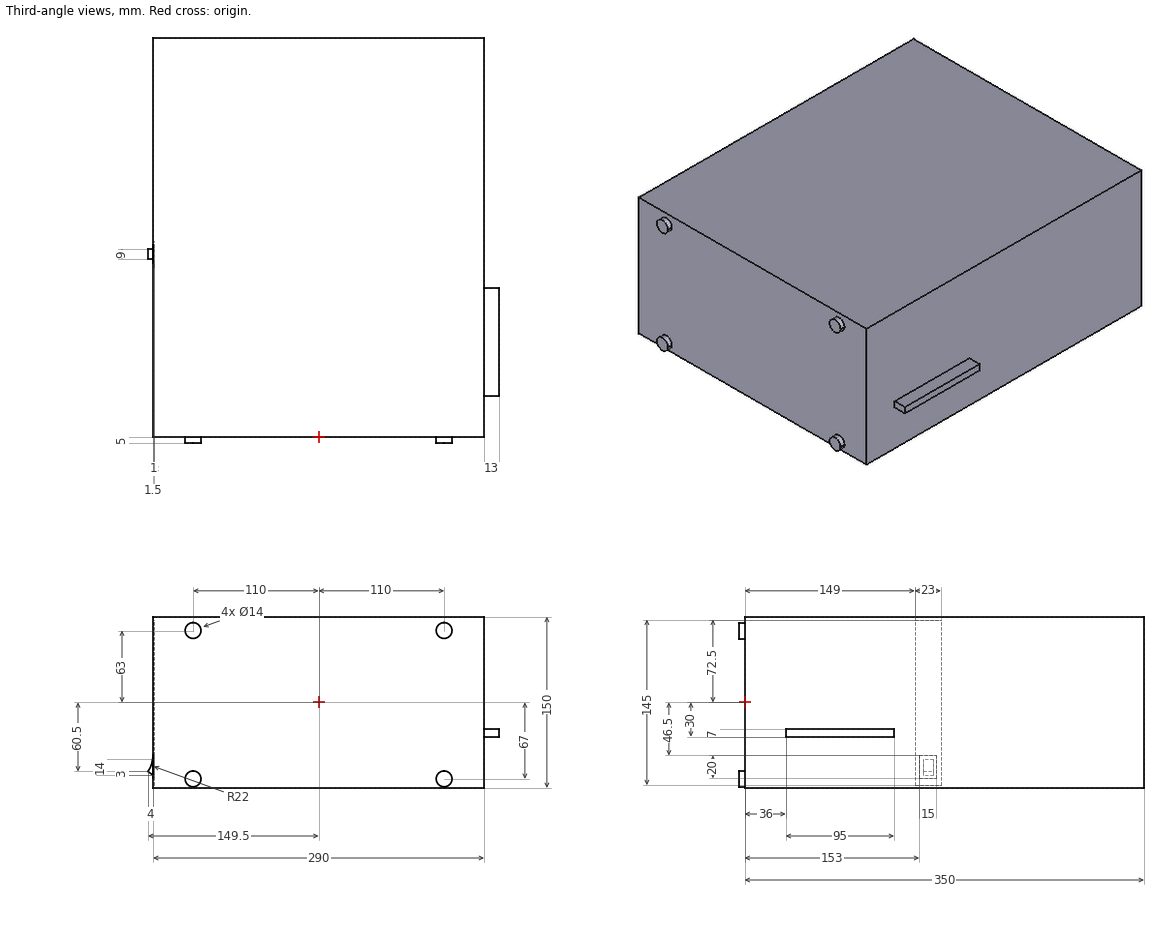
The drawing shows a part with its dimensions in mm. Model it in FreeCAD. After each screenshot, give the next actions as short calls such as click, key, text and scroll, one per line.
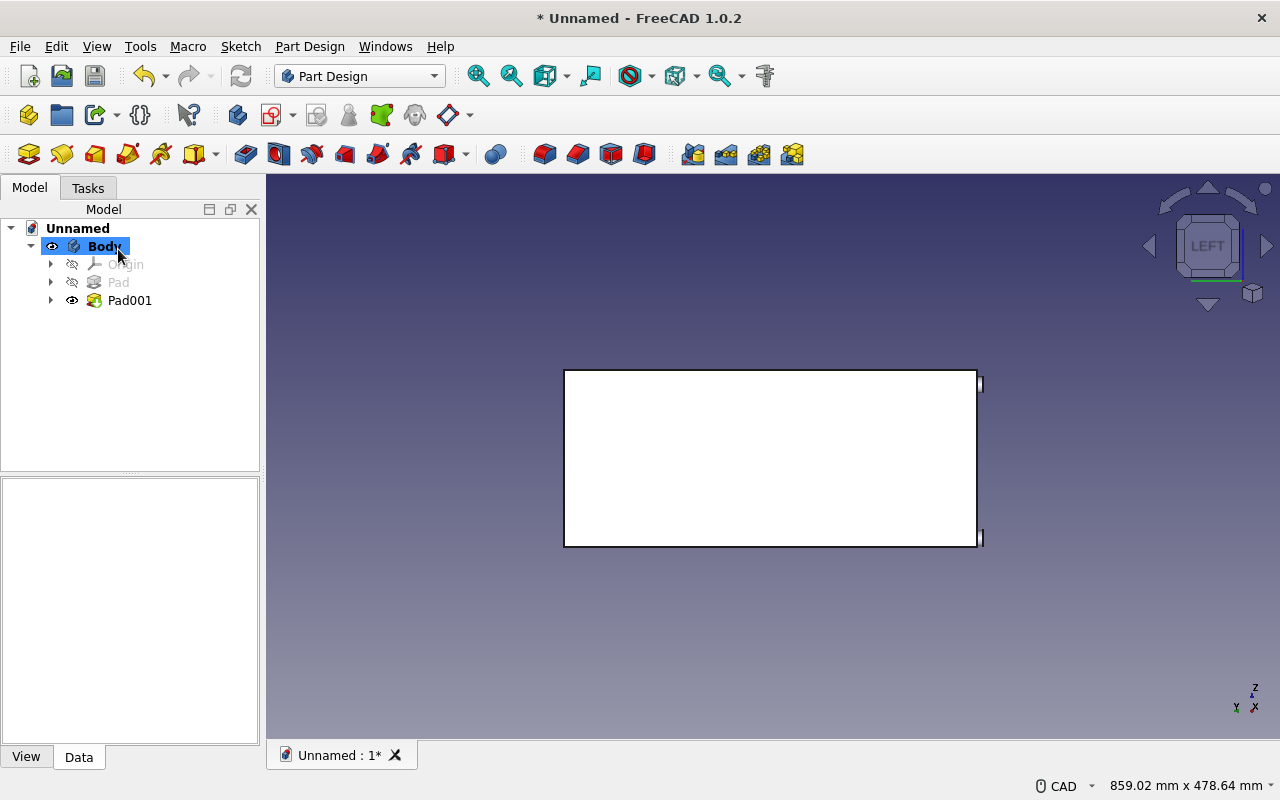
click(479, 76)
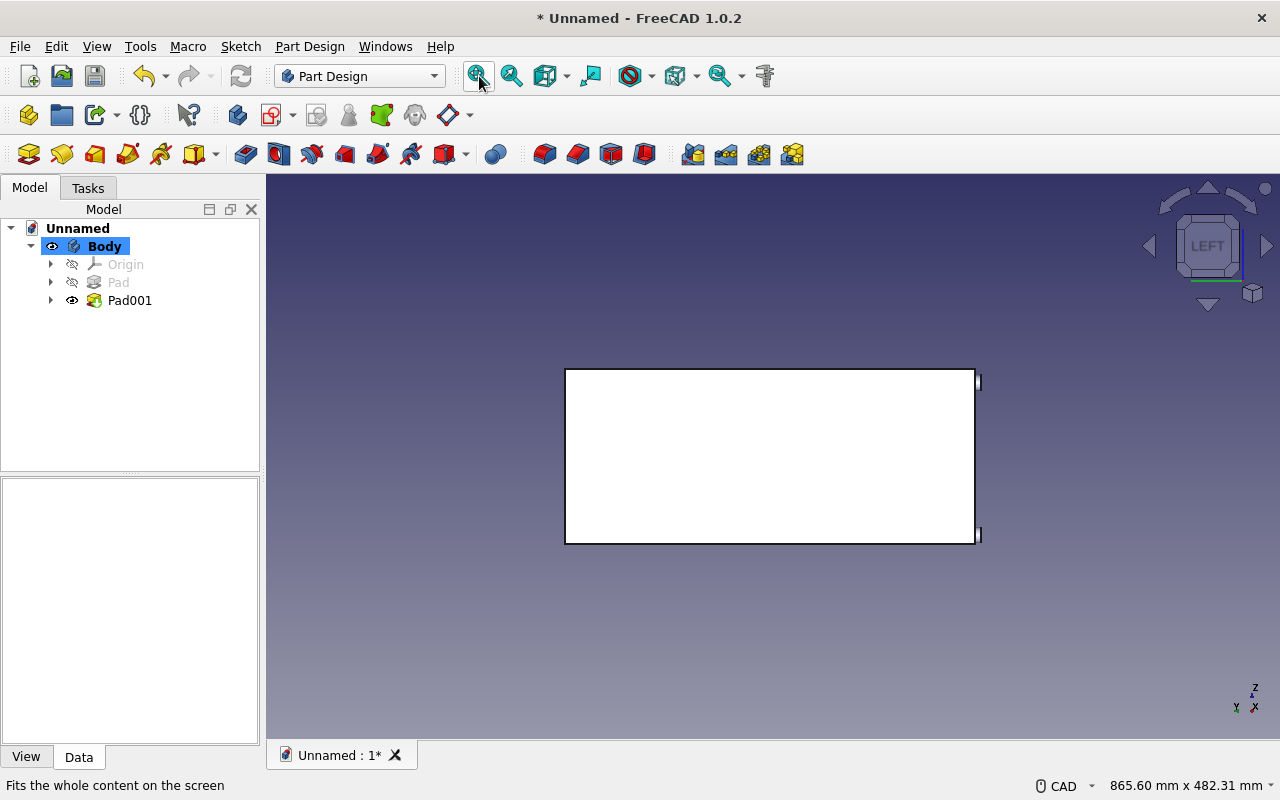
click(829, 456)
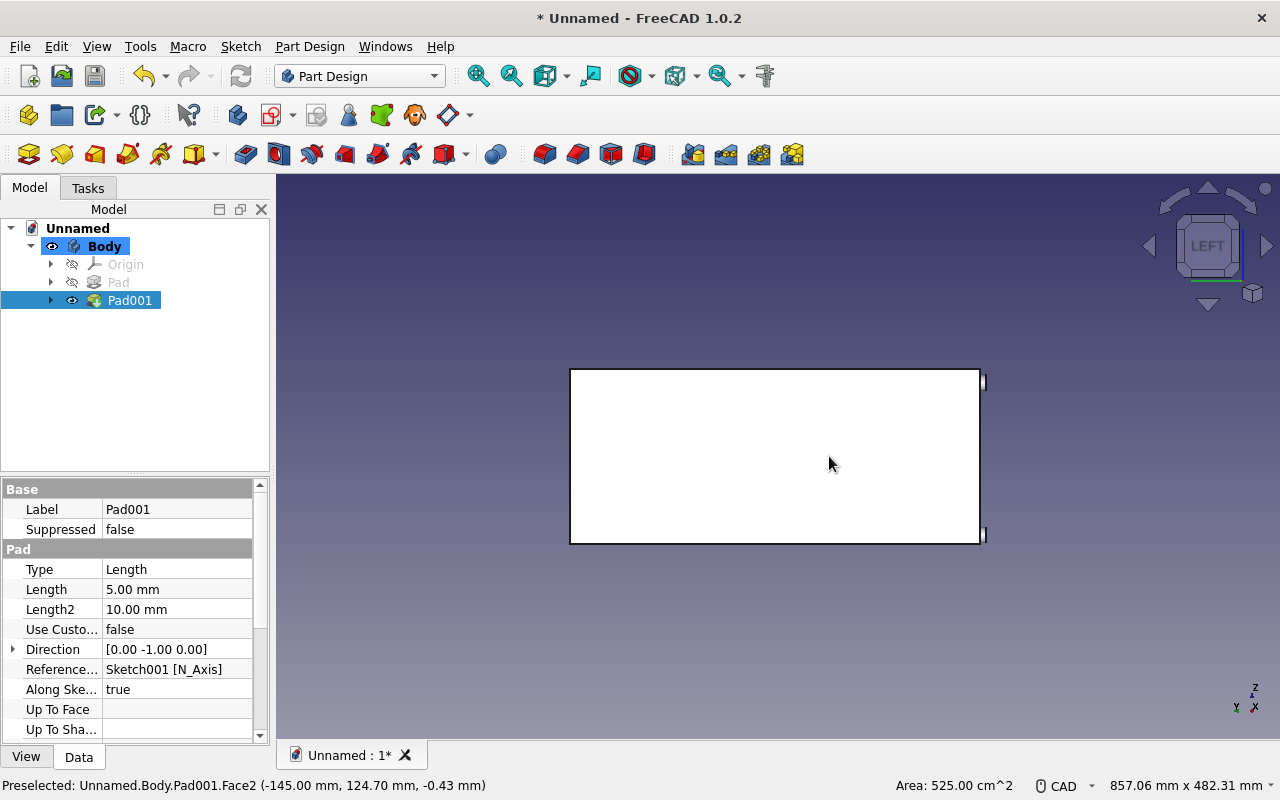
click(270, 116)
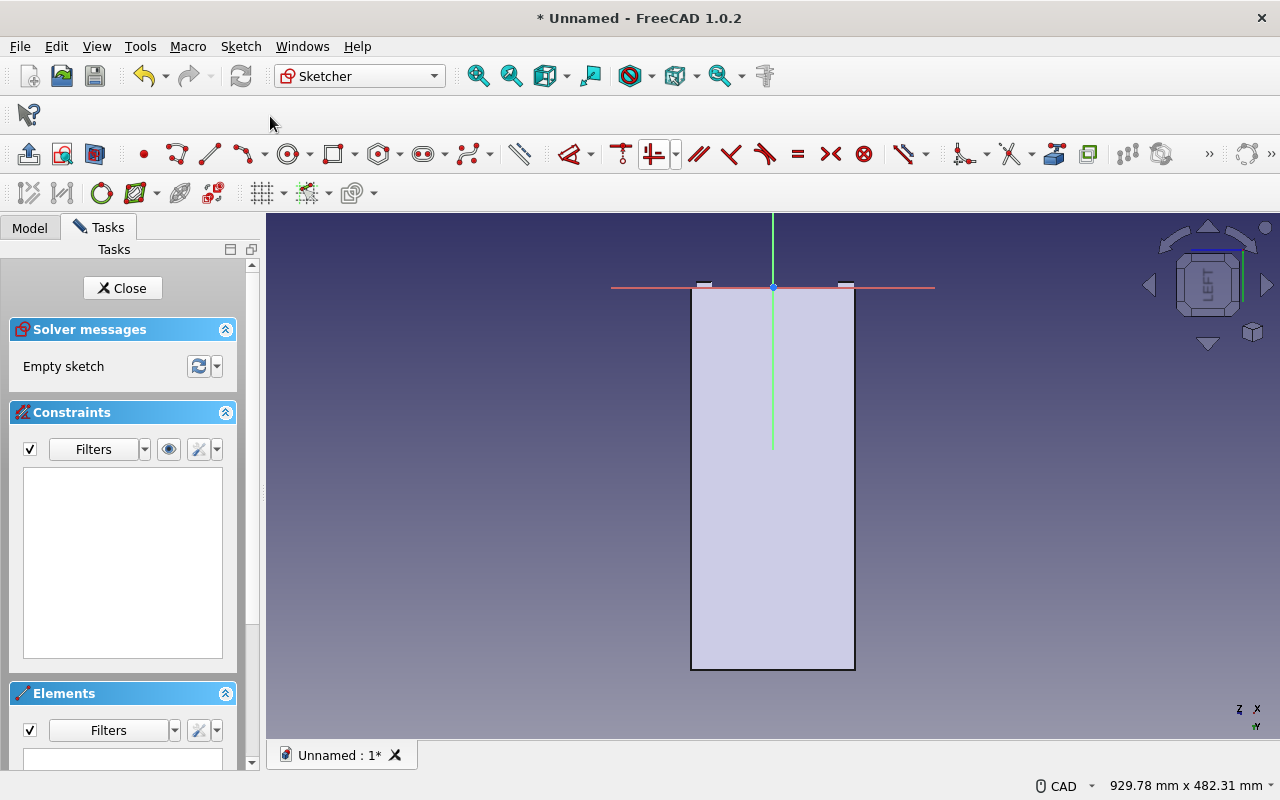
scroll(856, 267, up, 3)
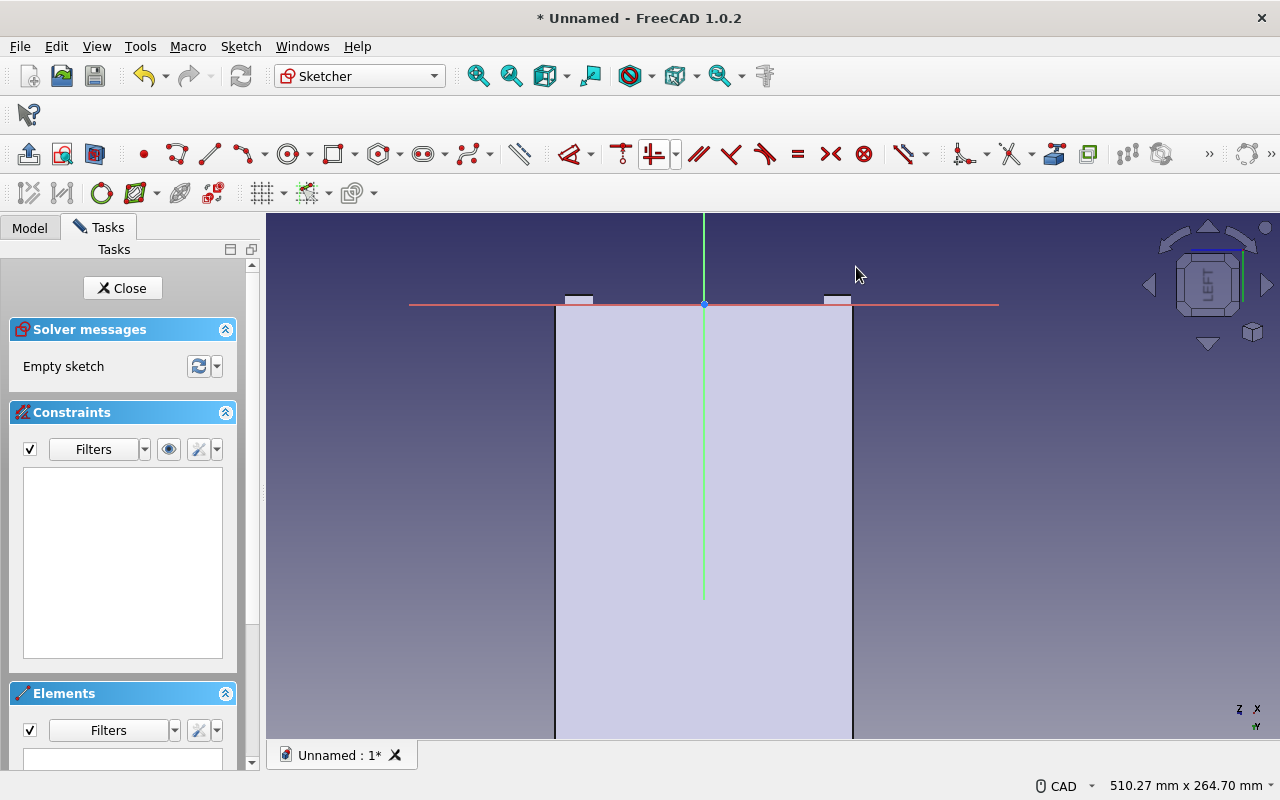
click(332, 154)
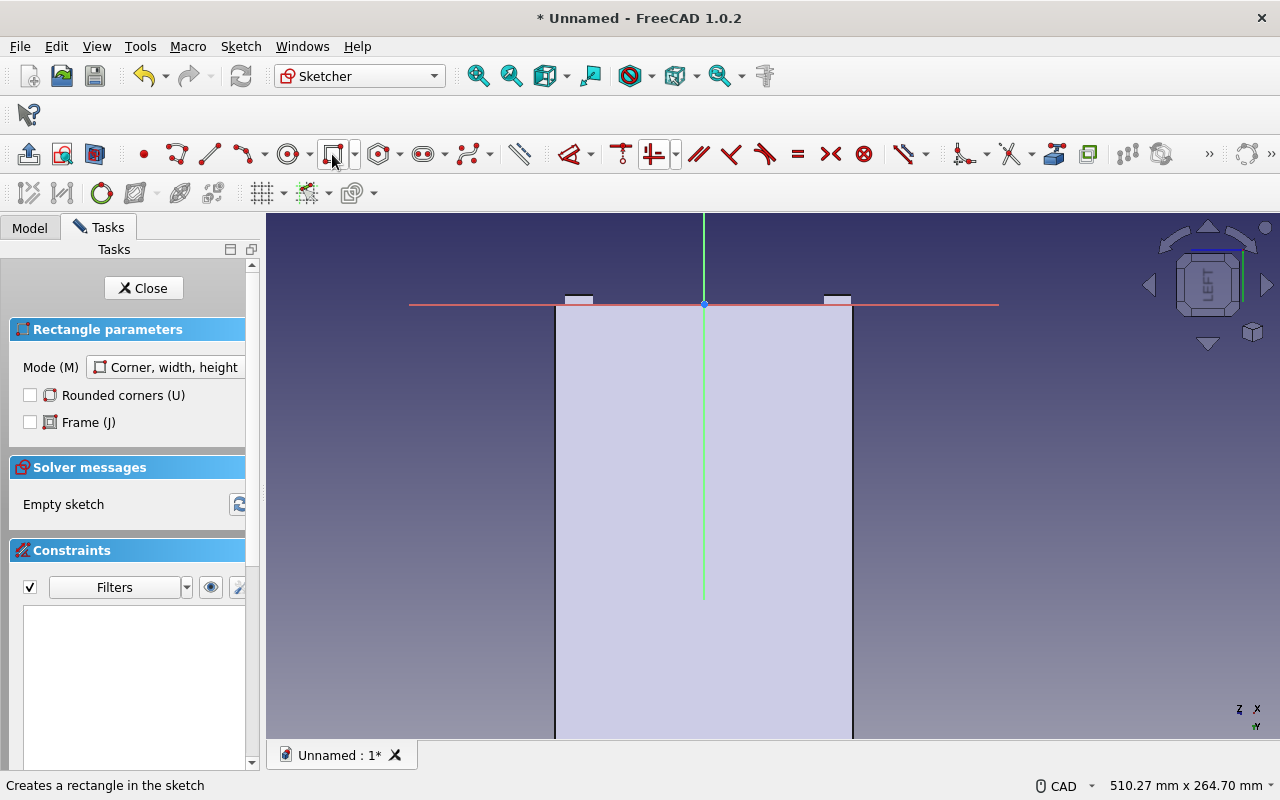
click(560, 601)
click(848, 647)
key(Escape)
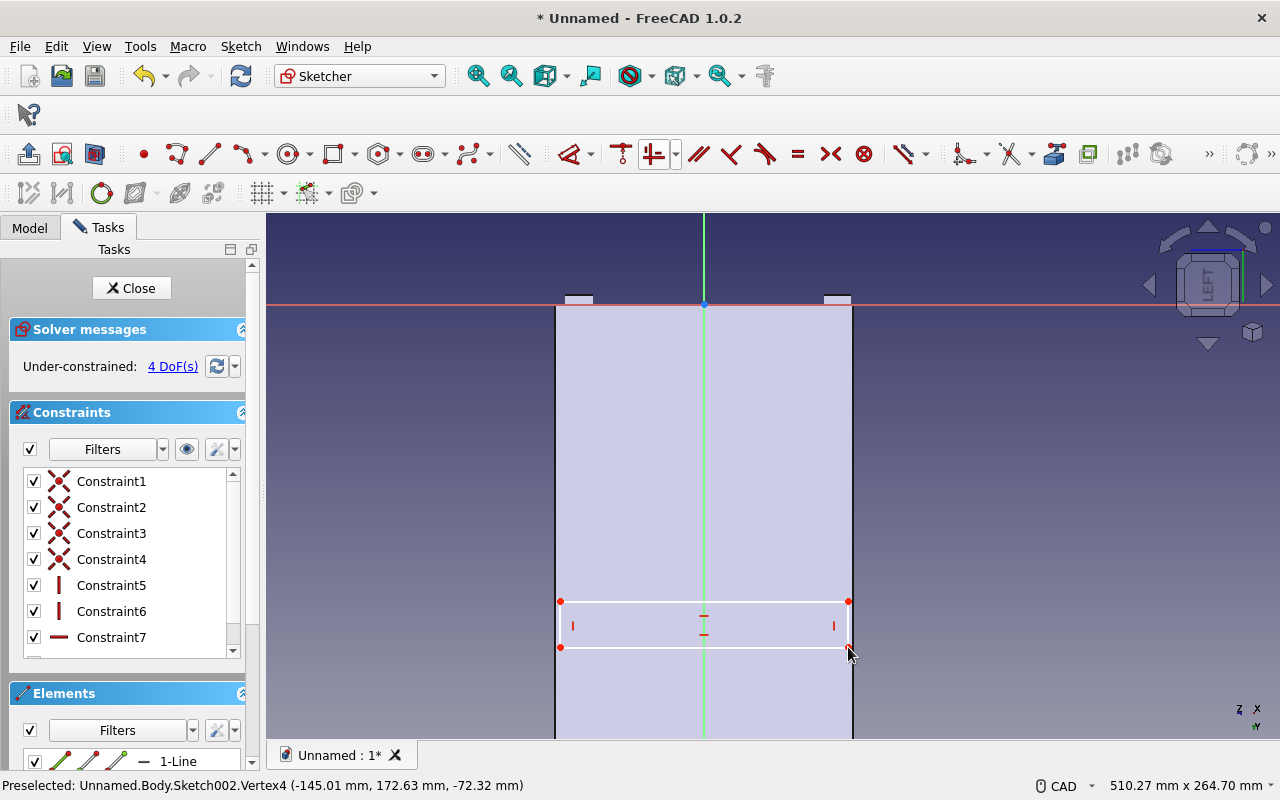
click(568, 154)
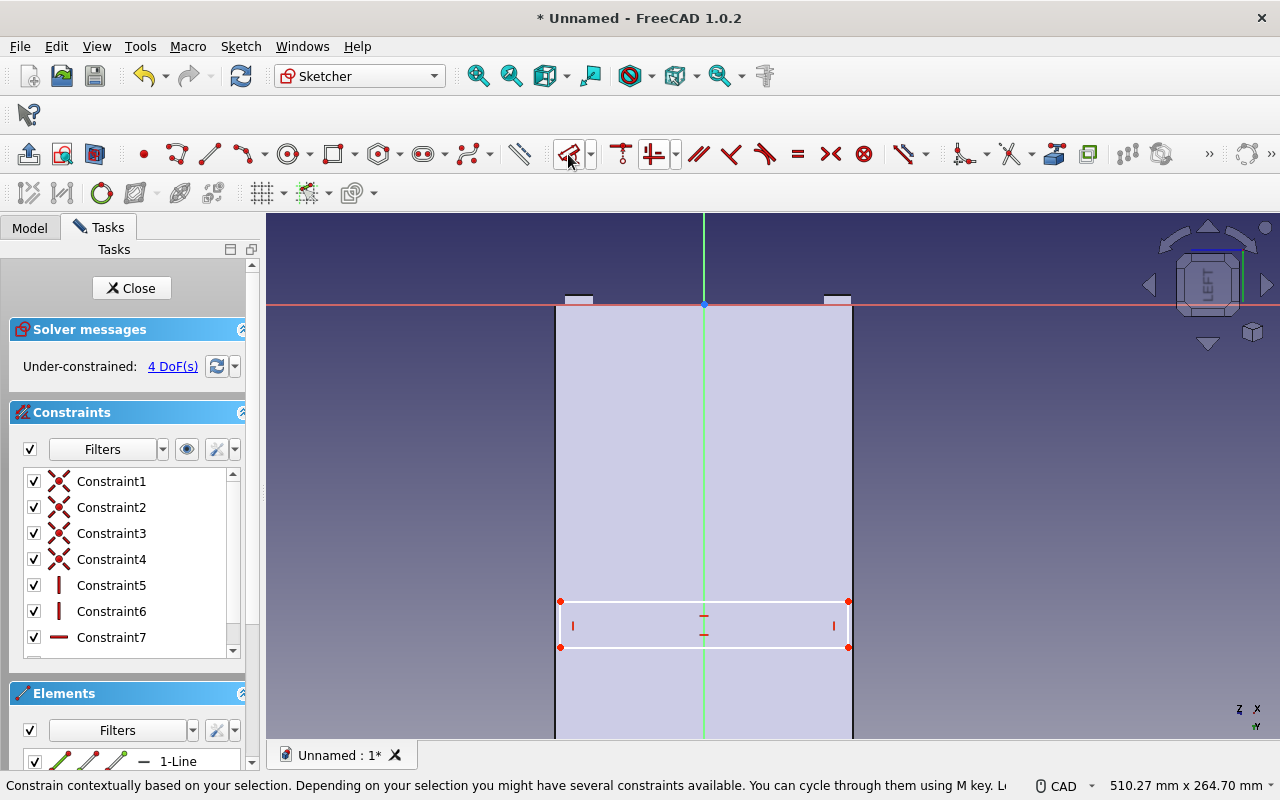
click(560, 616)
click(526, 625)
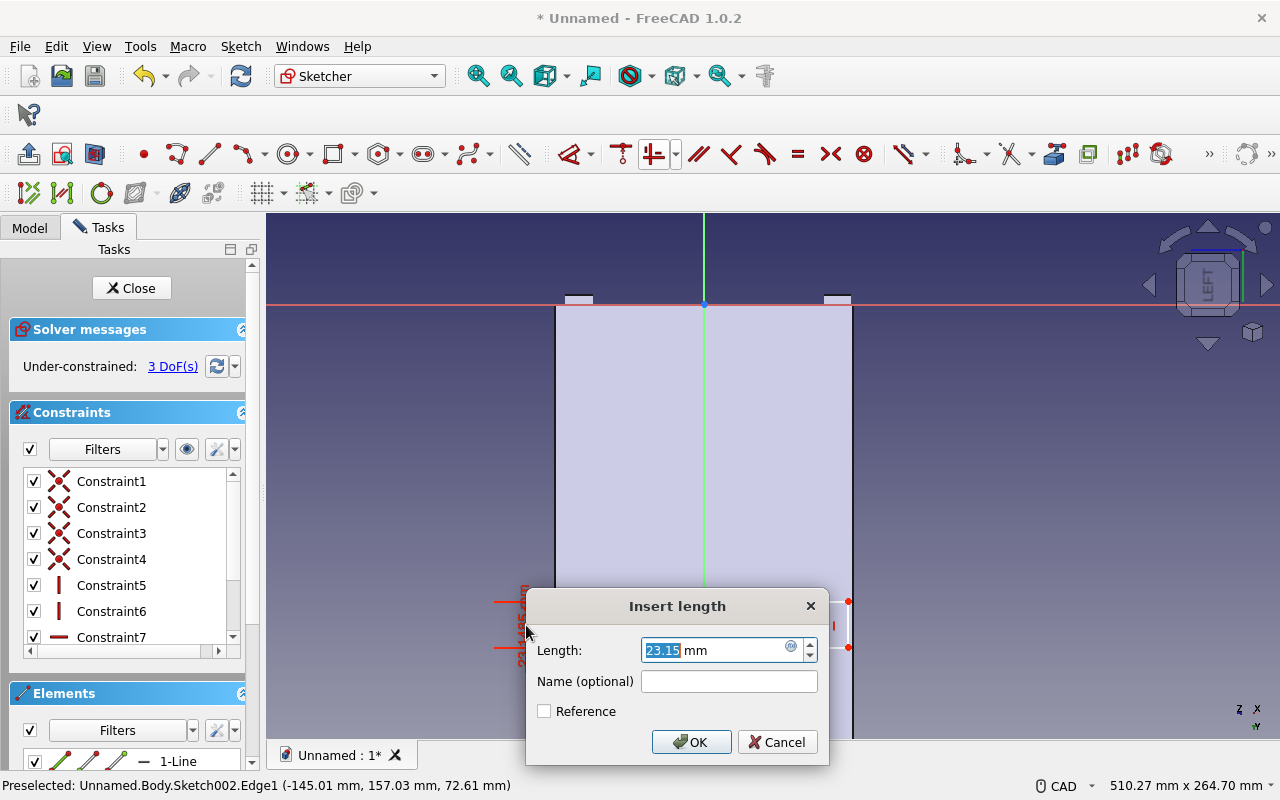
text(23)
key(Return)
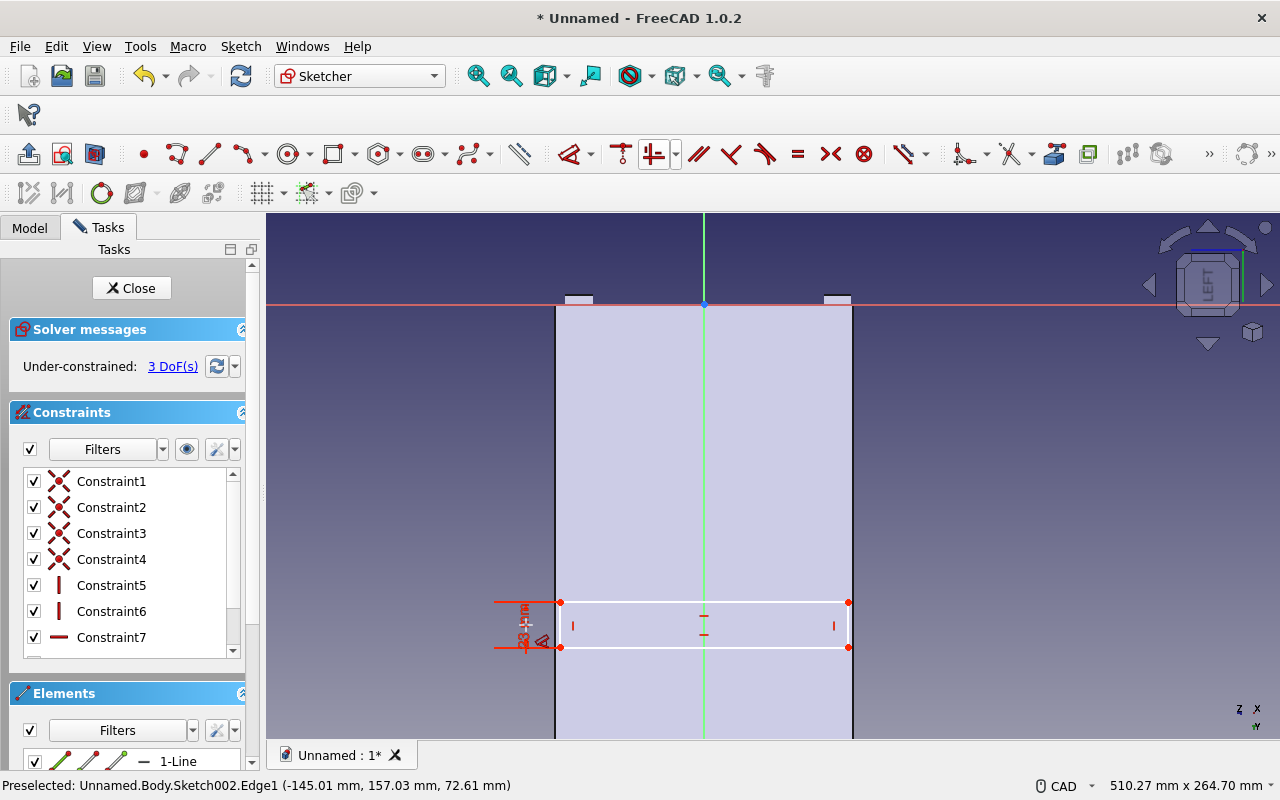
click(646, 648)
click(638, 682)